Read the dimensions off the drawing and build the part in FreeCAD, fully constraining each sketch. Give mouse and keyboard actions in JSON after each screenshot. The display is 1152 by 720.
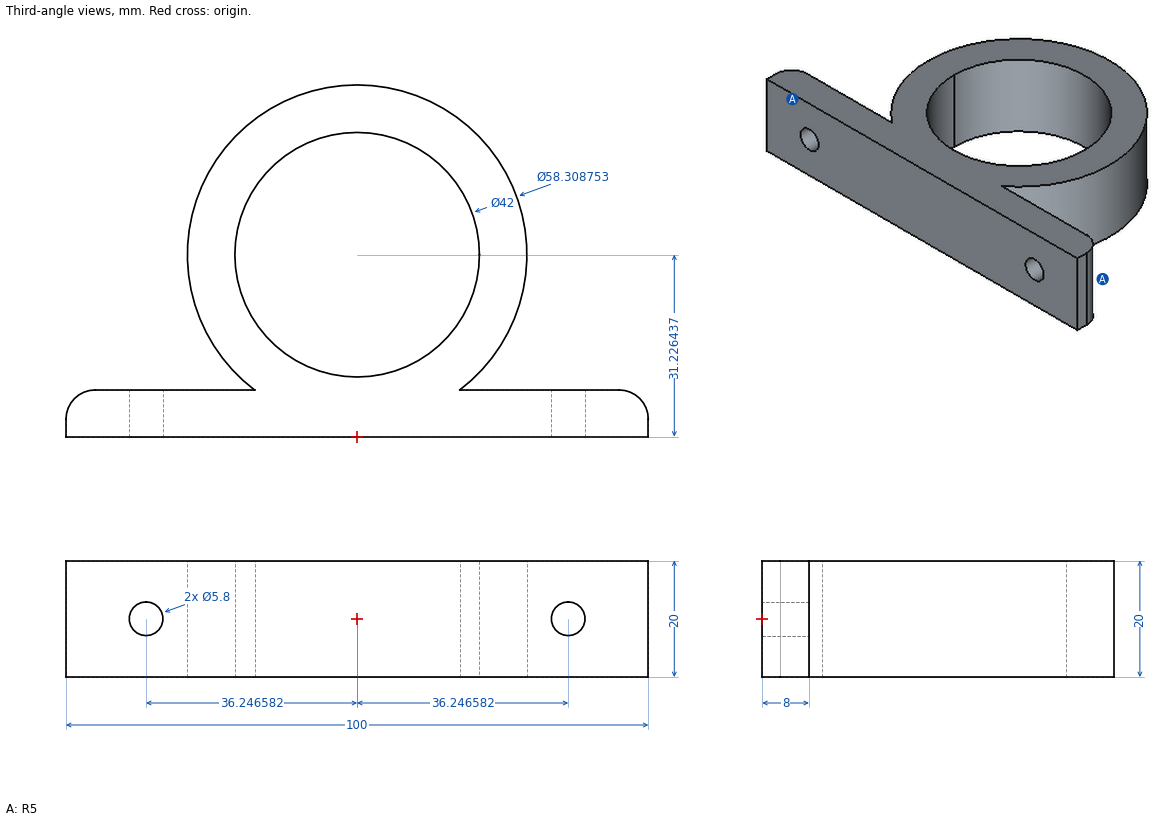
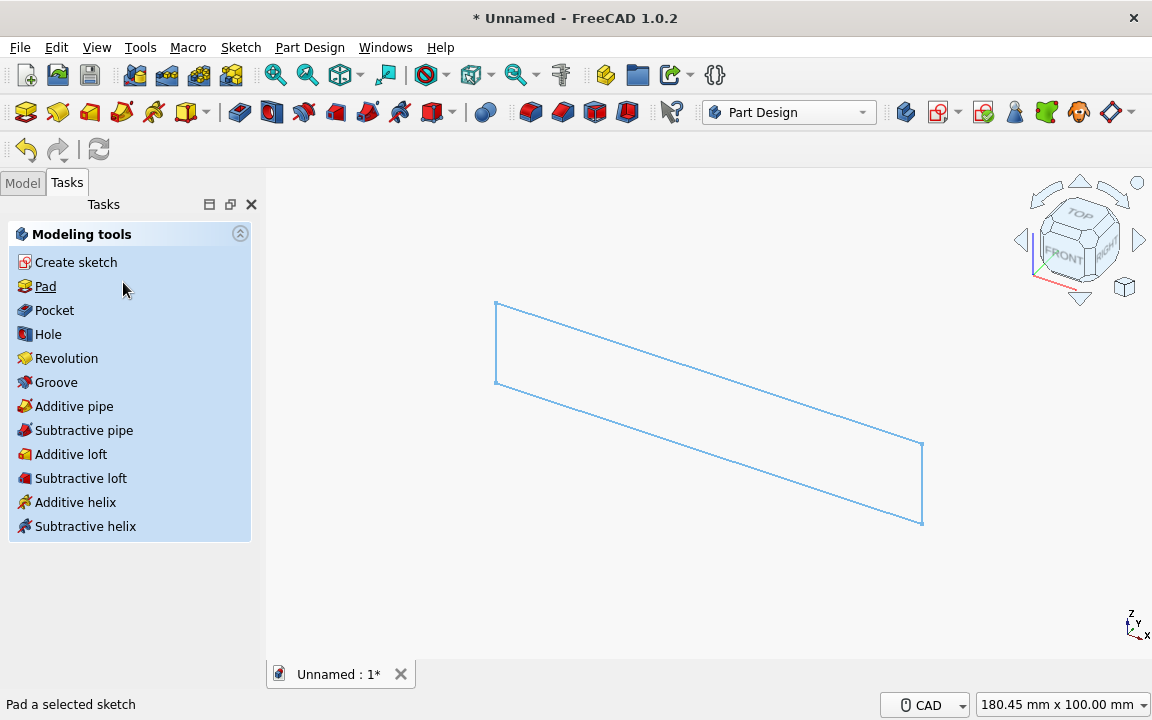
{"action": "left_click", "coordinate": [26, 112]}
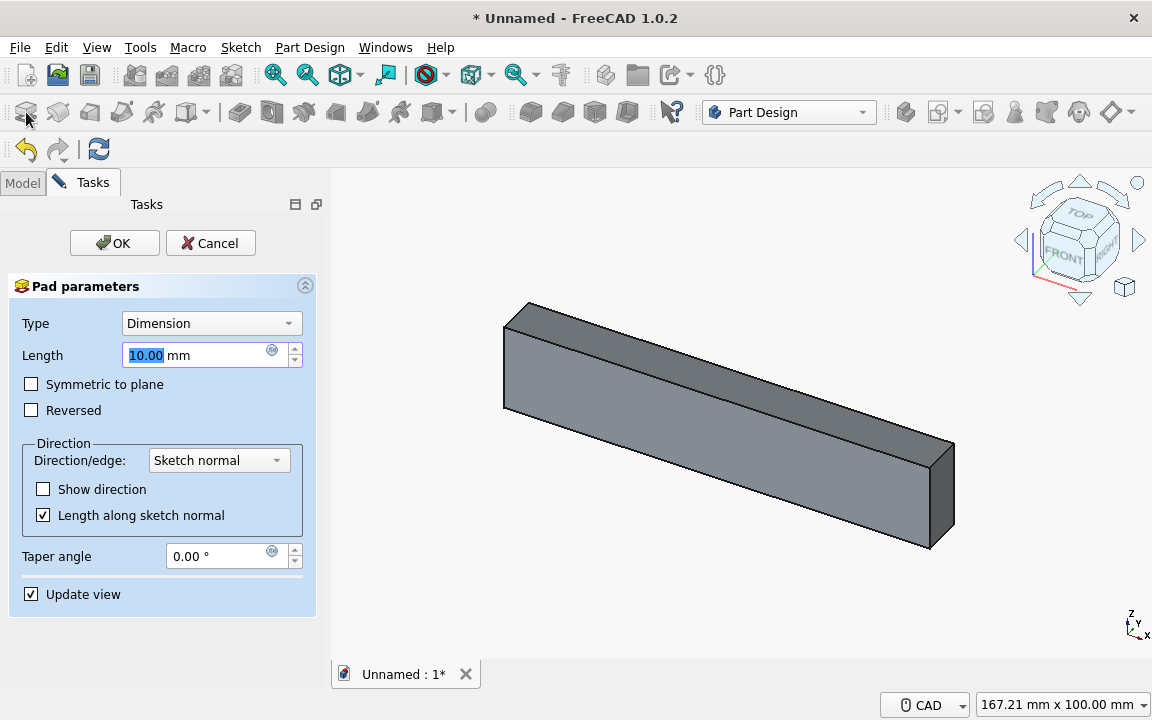
{"action": "type", "text": "8"}
{"action": "key", "text": "Tab"}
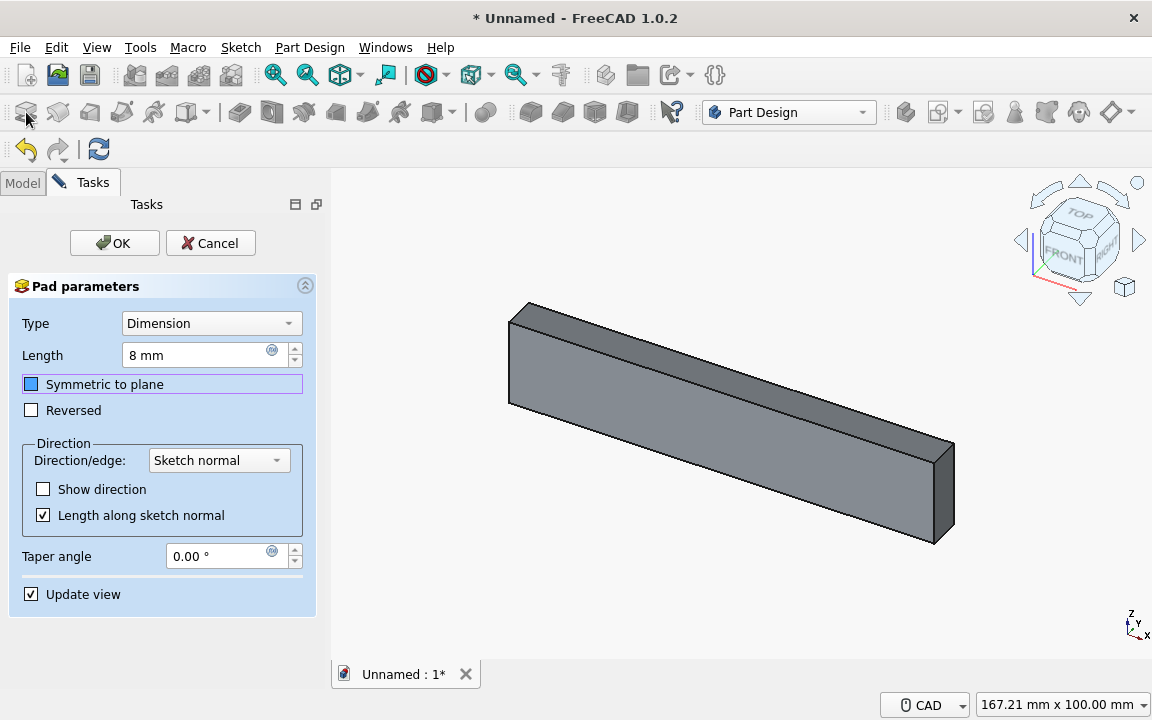
{"action": "left_click", "coordinate": [30, 410]}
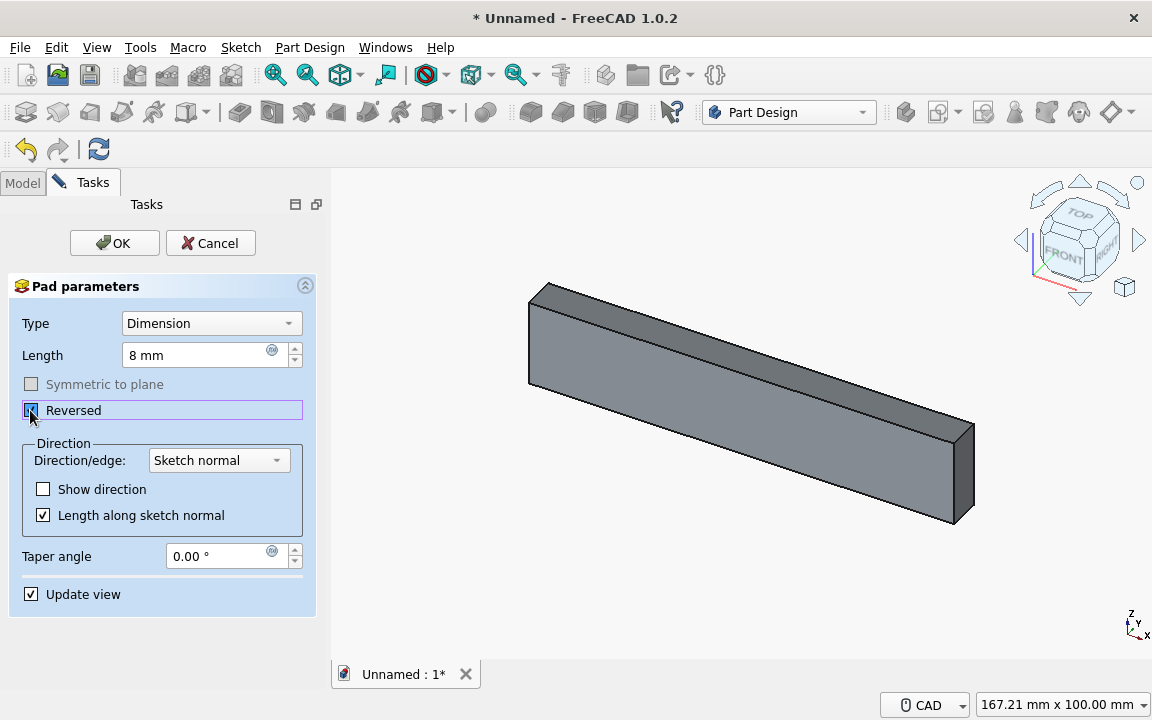
{"action": "left_click", "coordinate": [115, 243]}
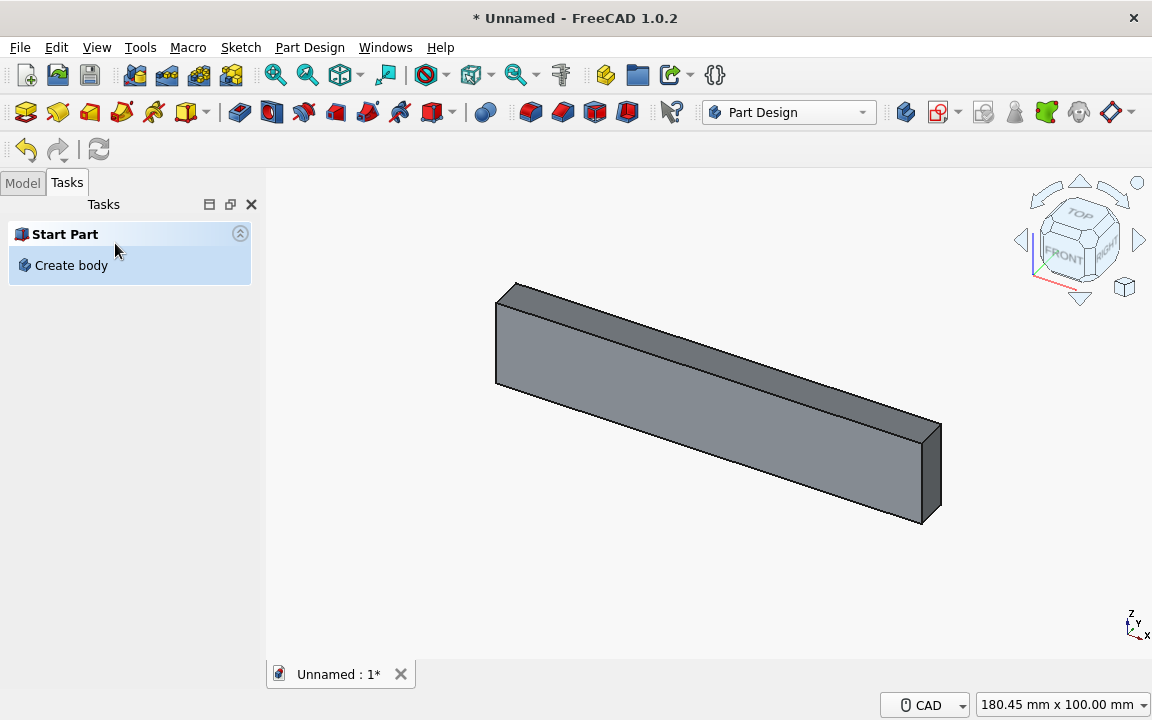
{"action": "key", "text": "0"}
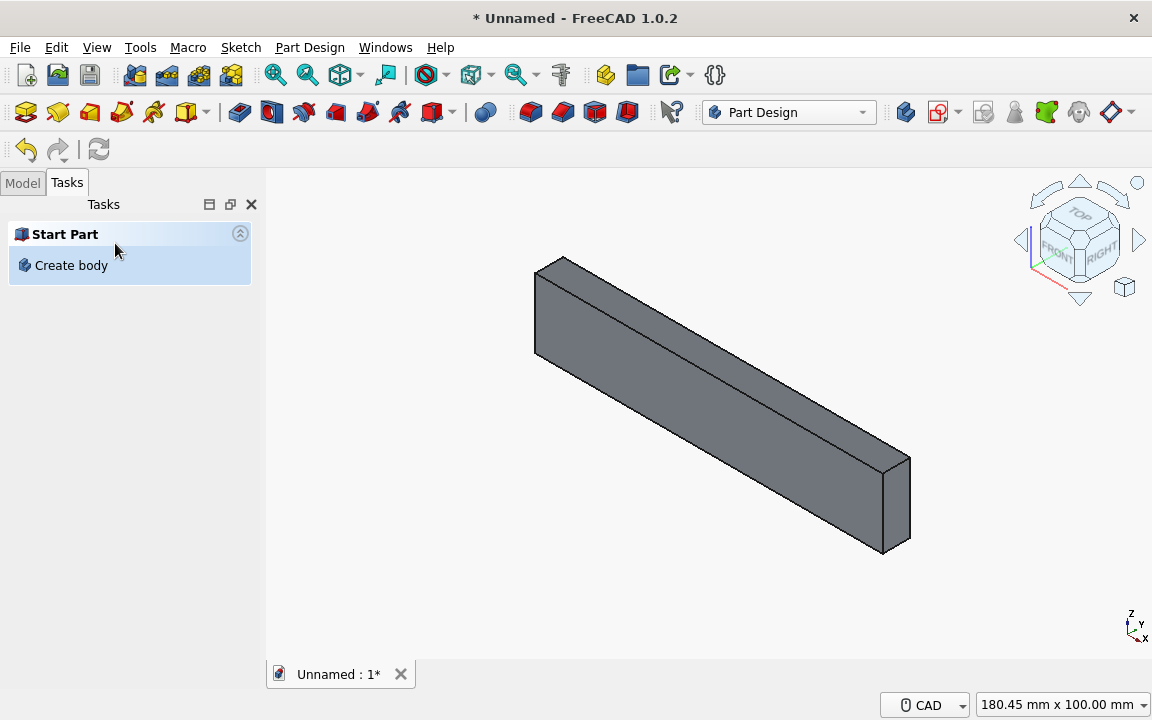
{"action": "key", "text": "2"}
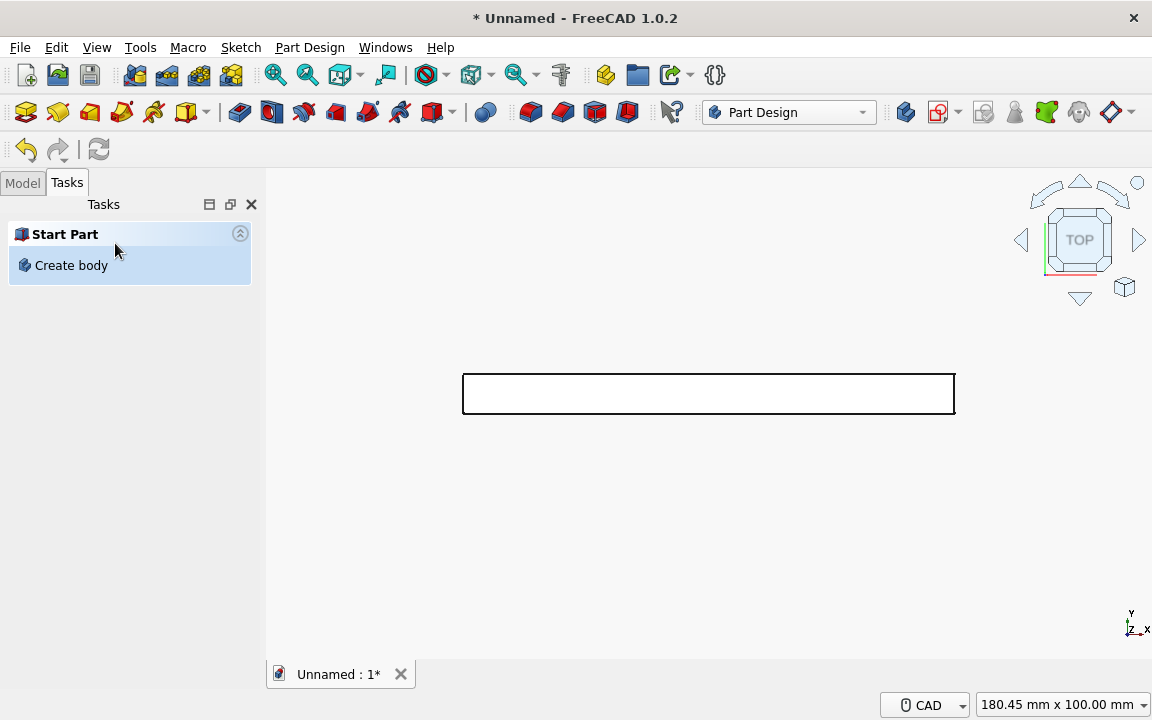
{"action": "key", "text": "1"}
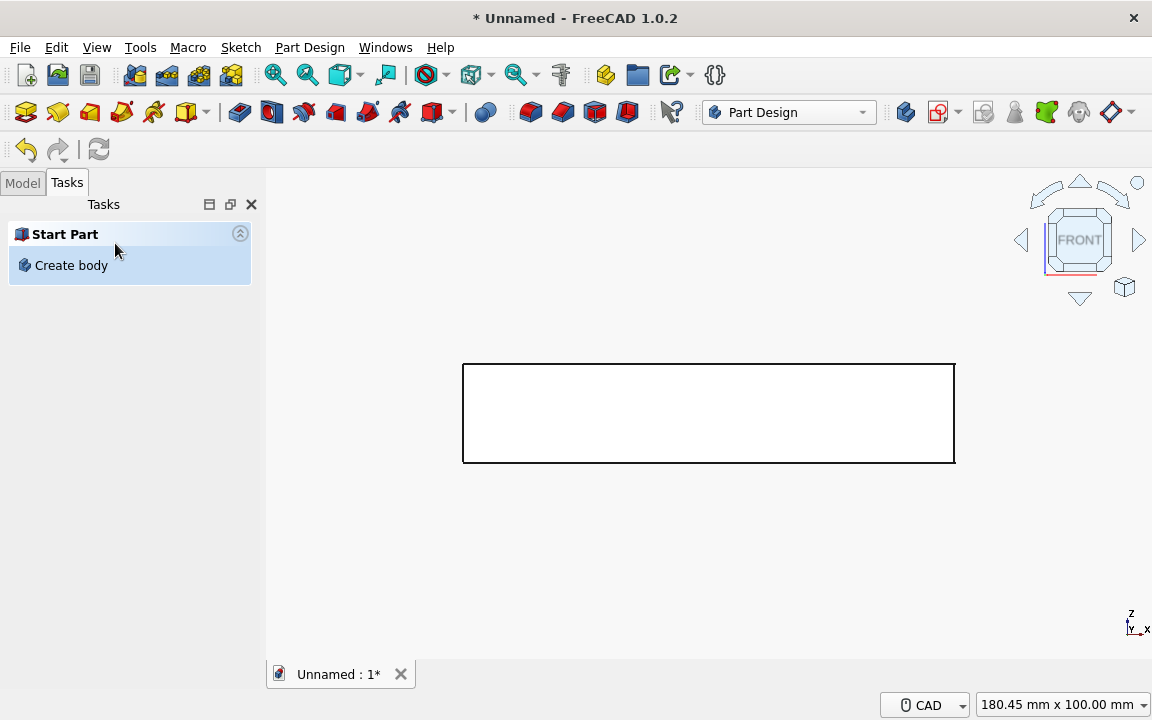
{"action": "key", "text": "3"}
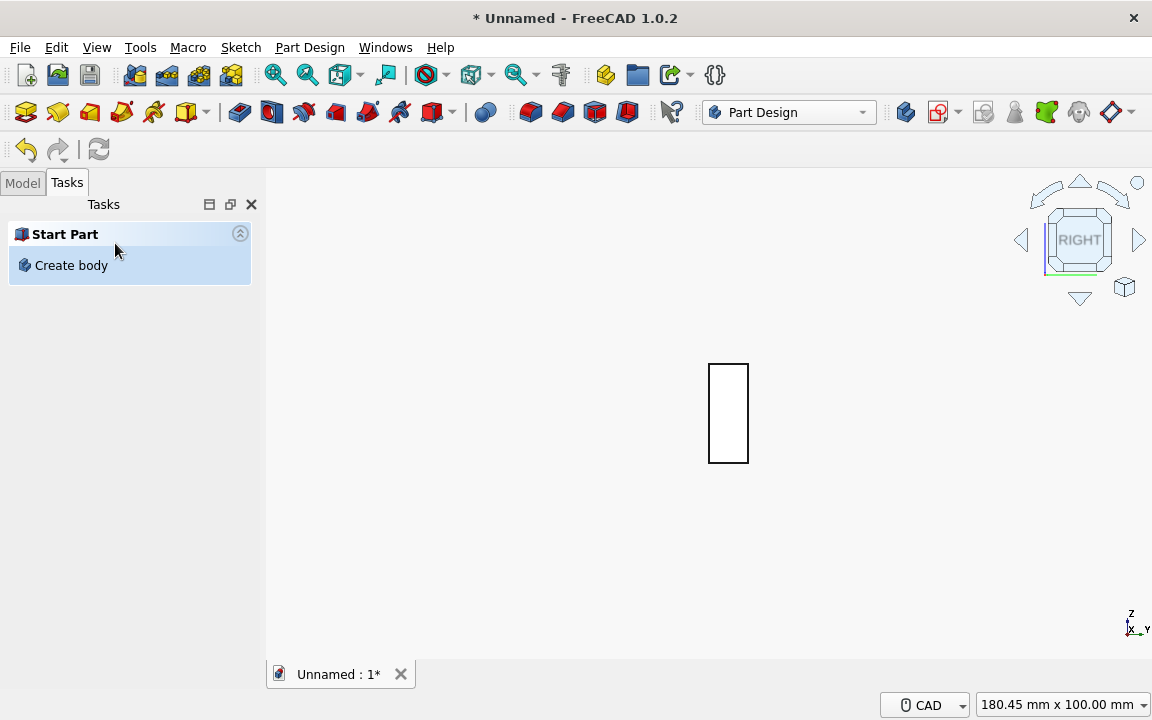
{"action": "left_click", "coordinate": [276, 76]}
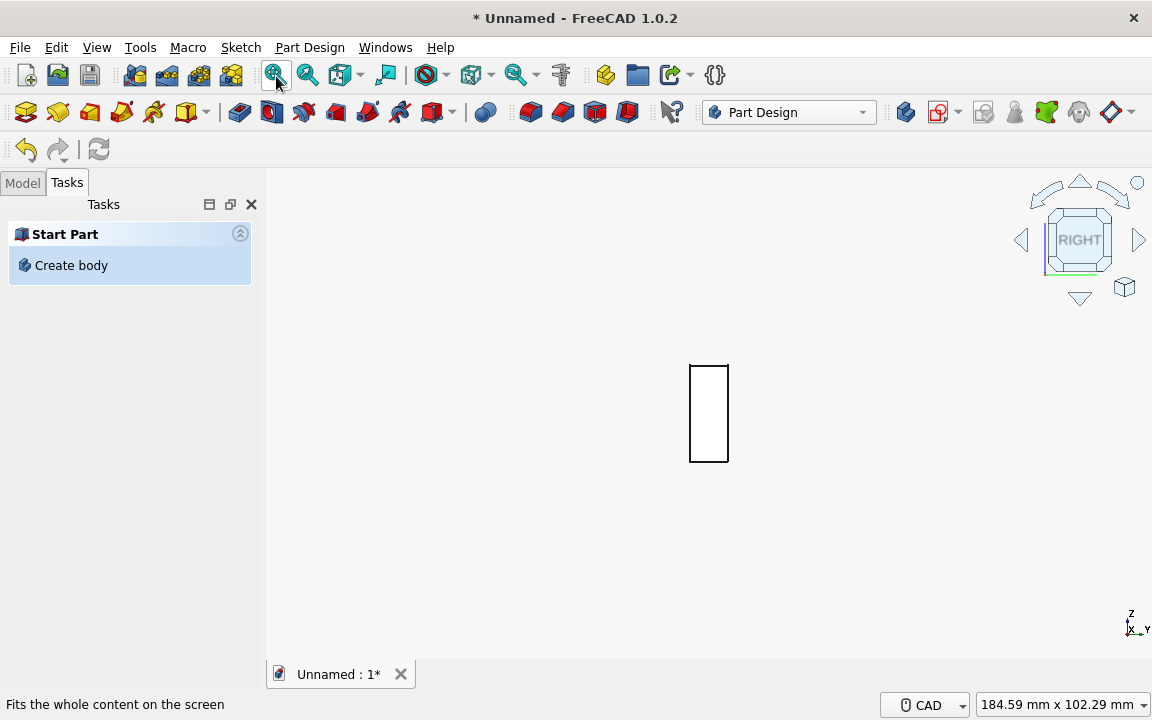
{"action": "left_click", "coordinate": [728, 412]}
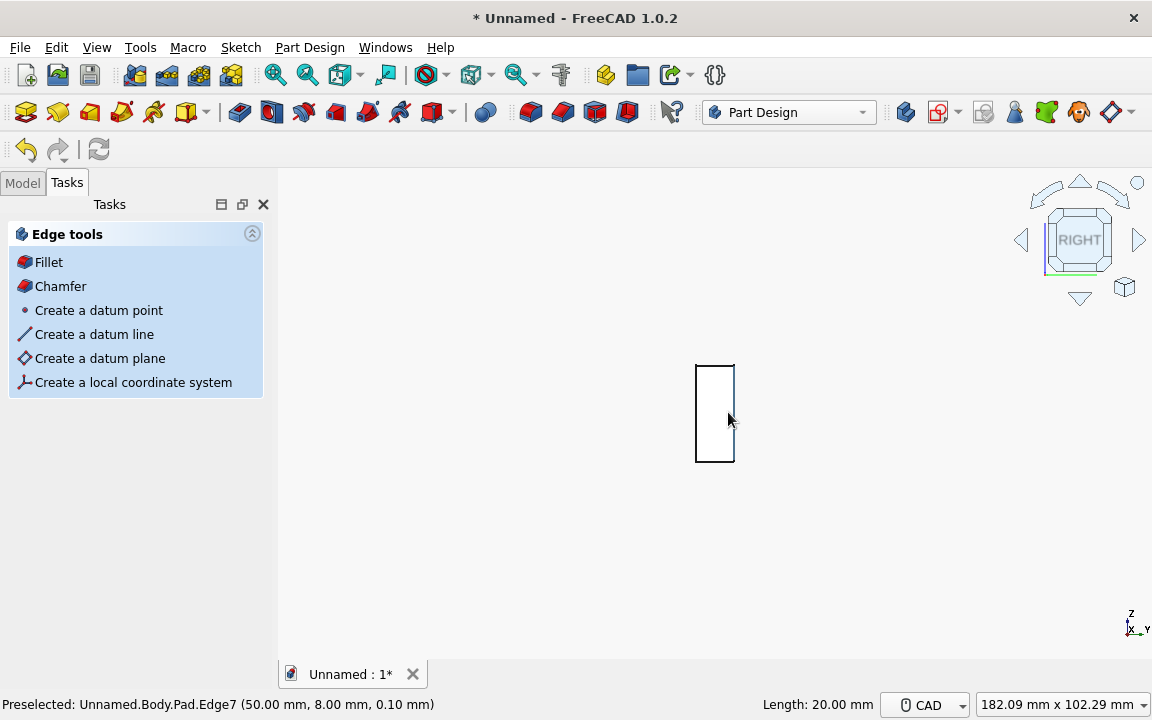
{"action": "key", "text": "5"}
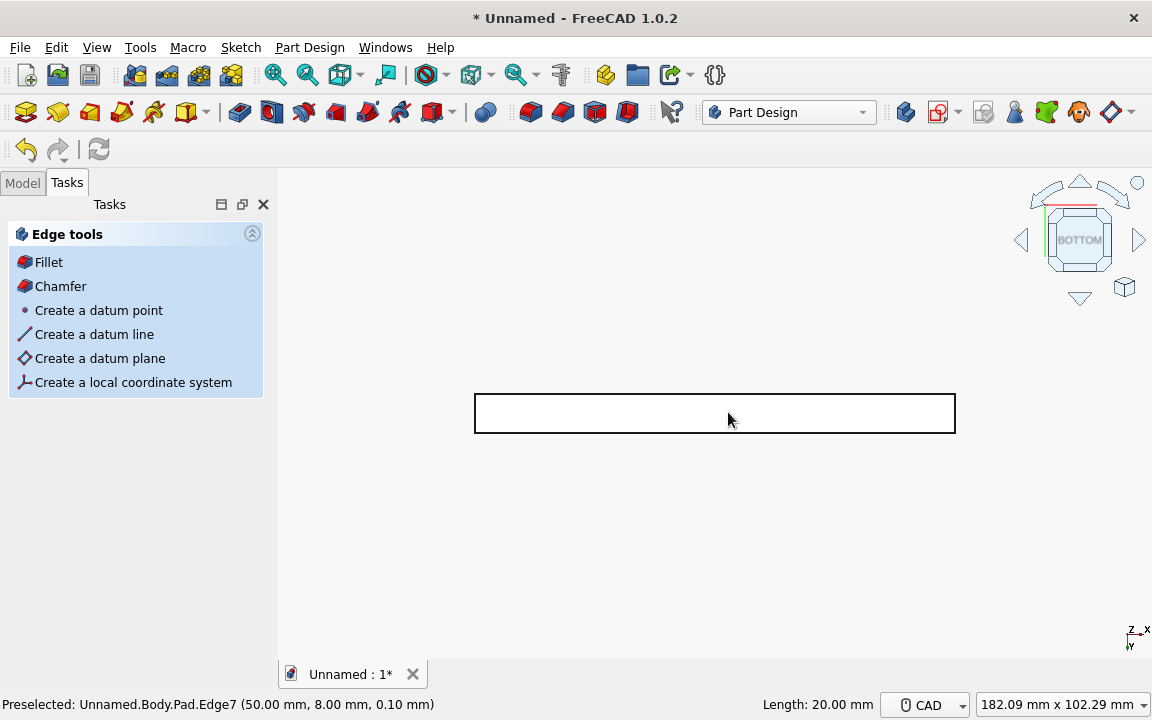
{"action": "key", "text": "4"}